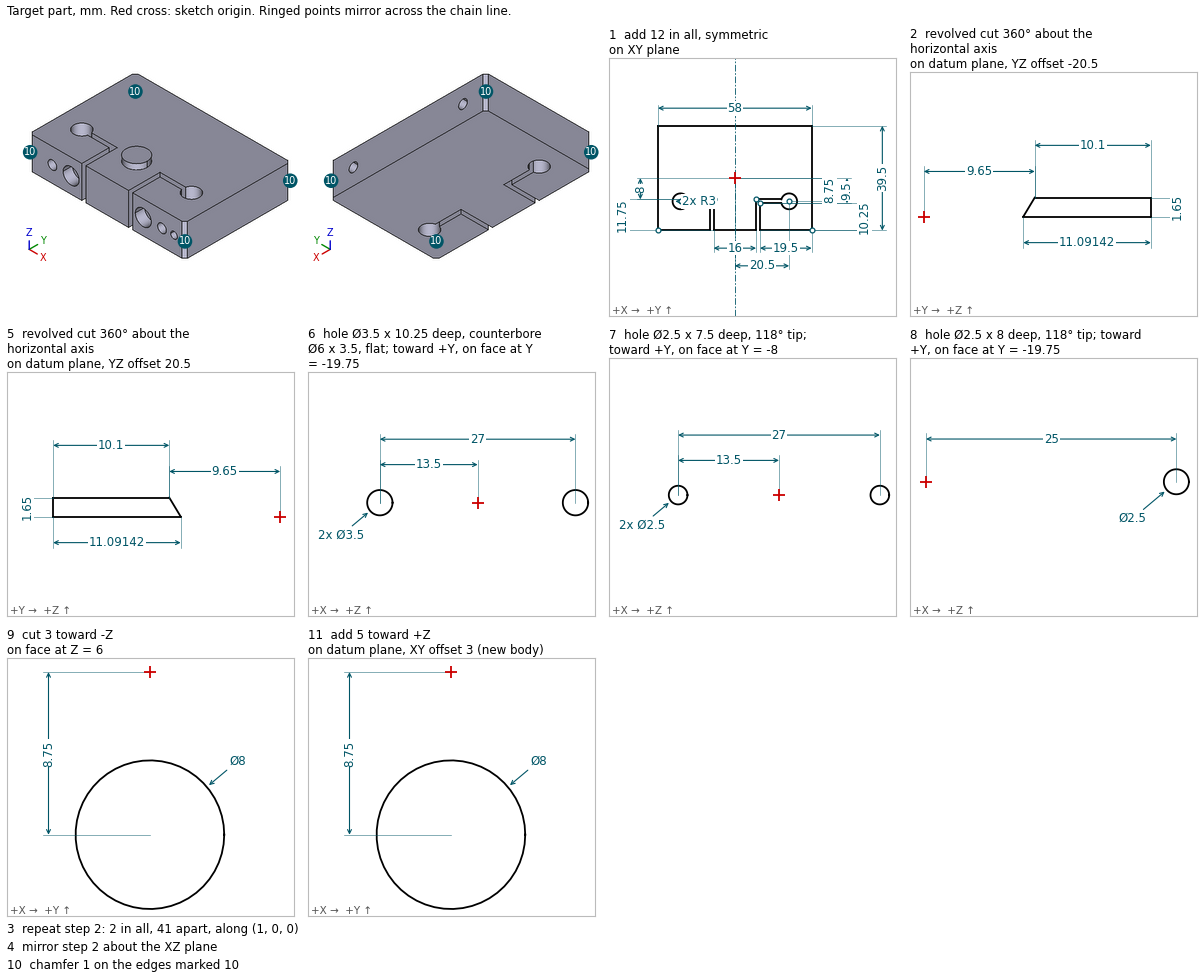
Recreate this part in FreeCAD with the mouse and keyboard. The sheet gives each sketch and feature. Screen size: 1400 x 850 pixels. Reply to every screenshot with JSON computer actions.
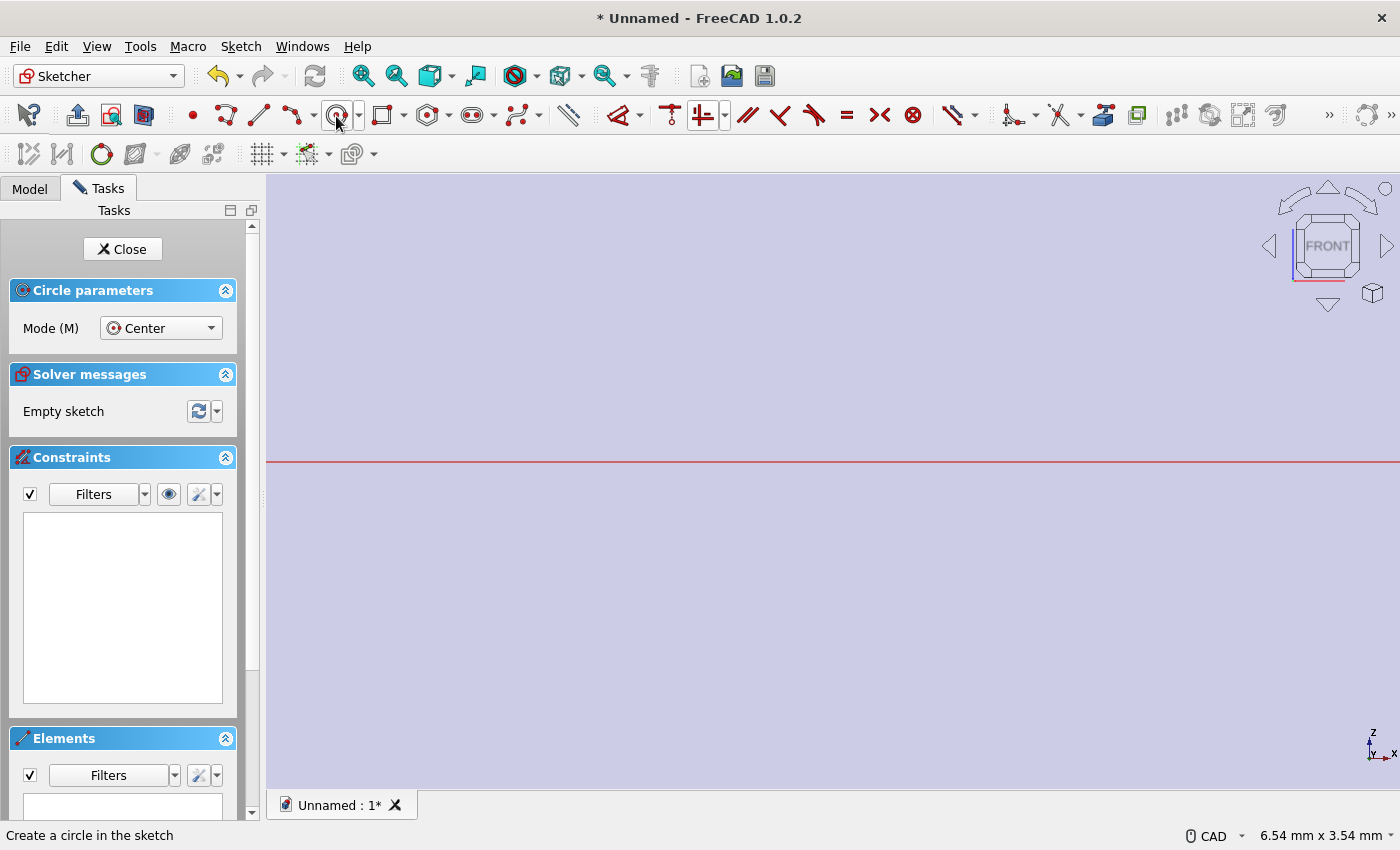
{"action": "left_click", "coordinate": [749, 462]}
{"action": "left_click", "coordinate": [902, 309]}
{"action": "key", "text": "Escape"}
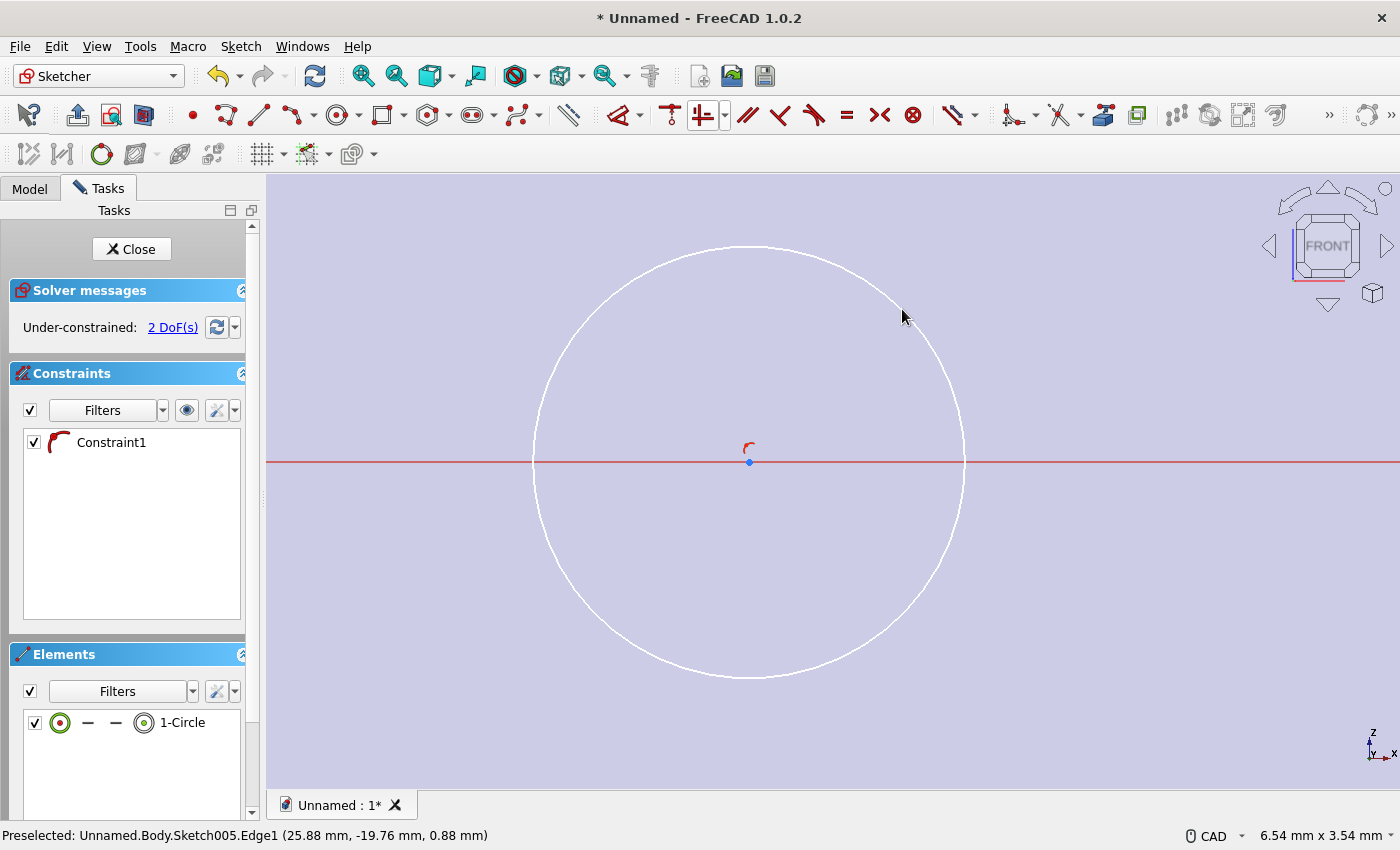
{"action": "left_click", "coordinate": [618, 116]}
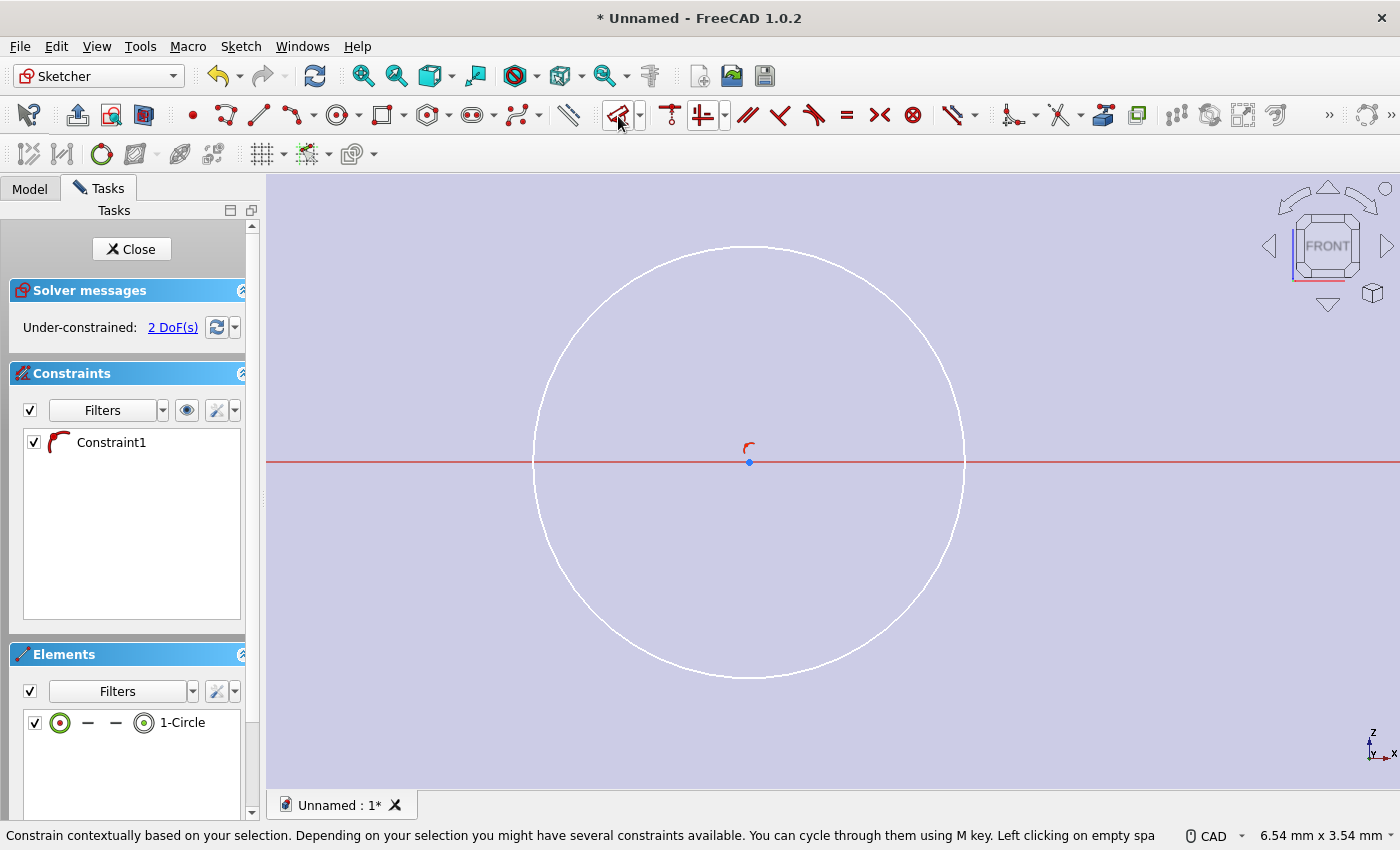
{"action": "left_click", "coordinate": [901, 309]}
{"action": "left_click", "coordinate": [924, 286]}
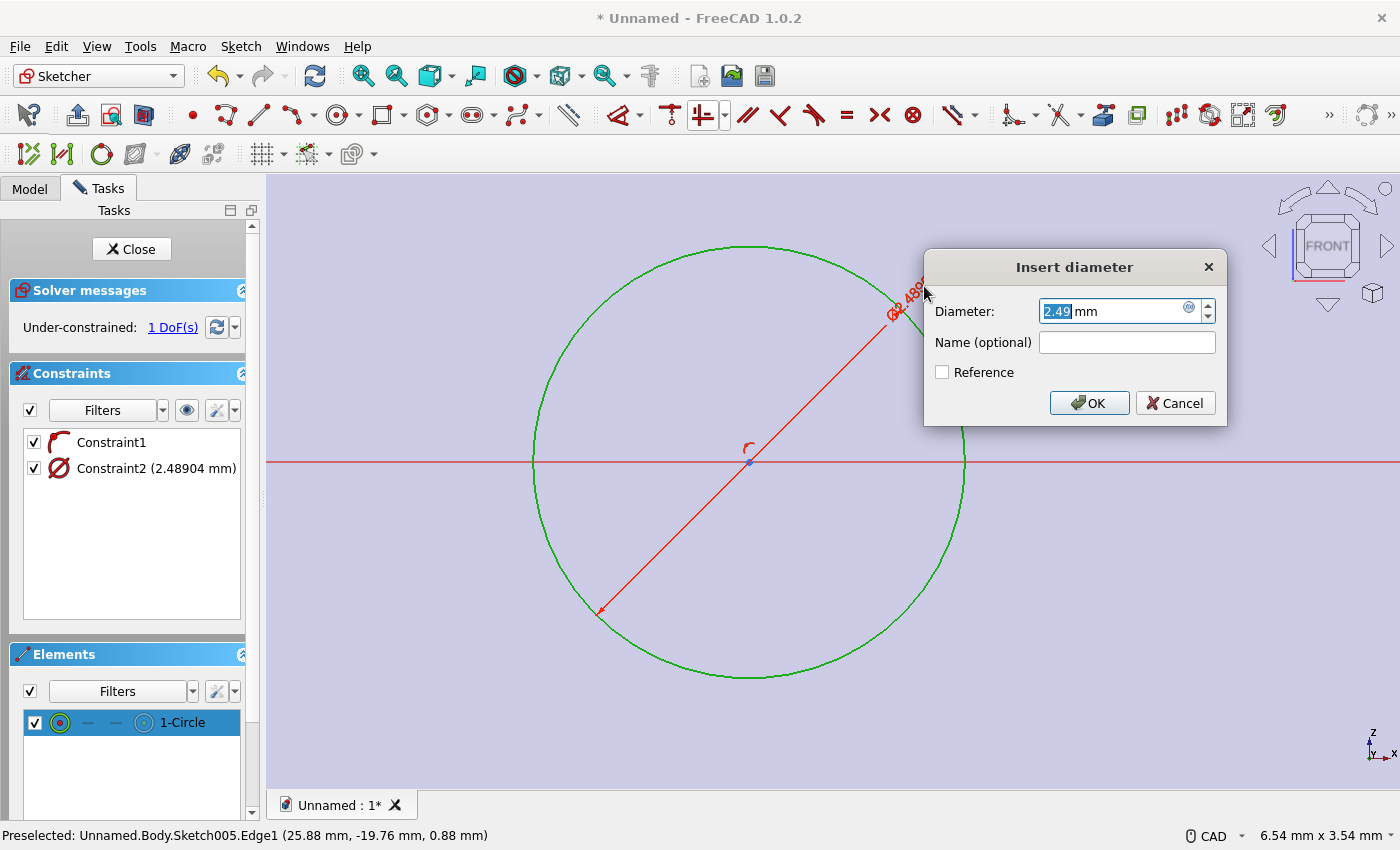
{"action": "type", "text": "2.5"}
{"action": "key", "text": "Return"}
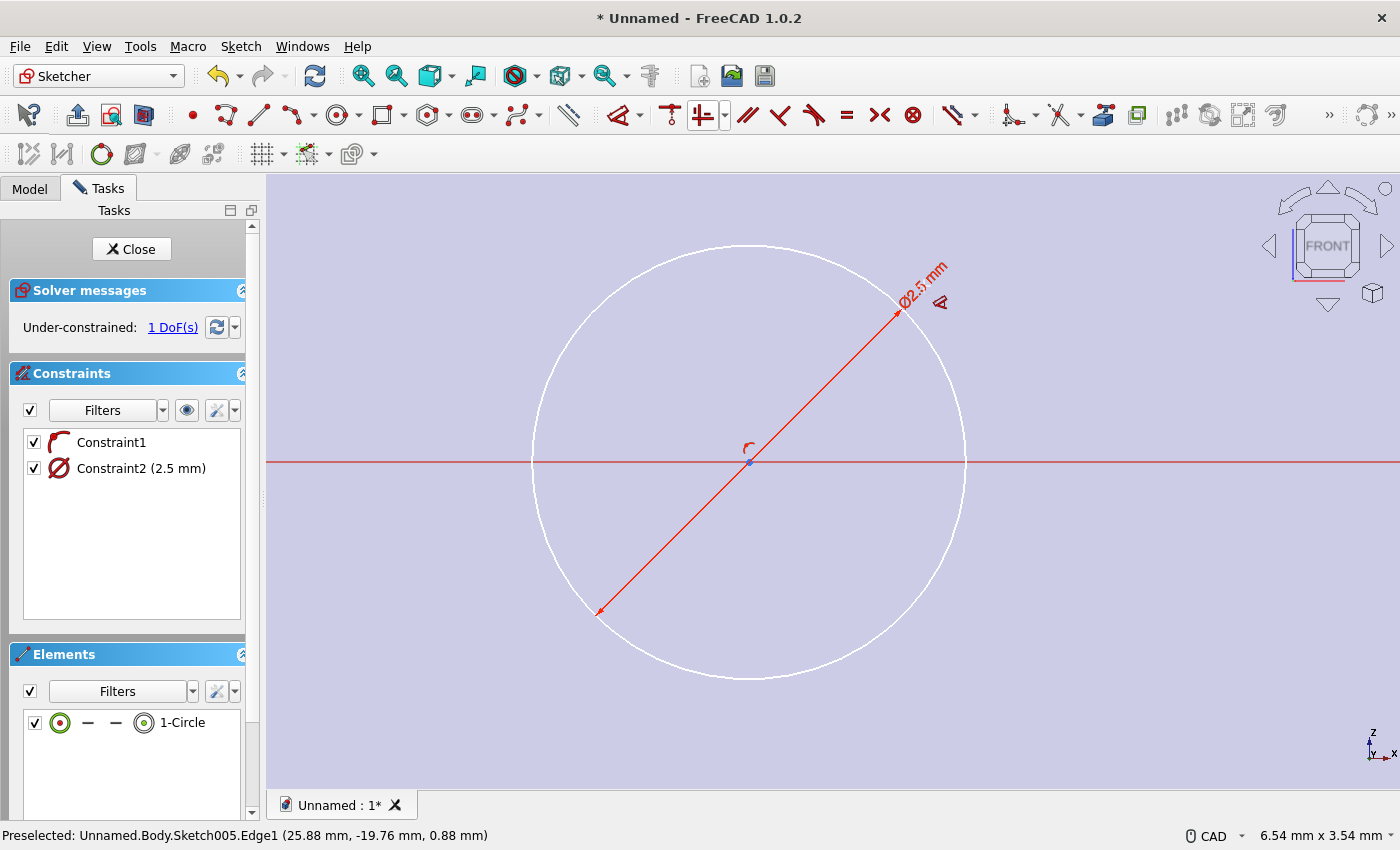
{"action": "left_click", "coordinate": [749, 462]}
{"action": "left_click", "coordinate": [522, 496]}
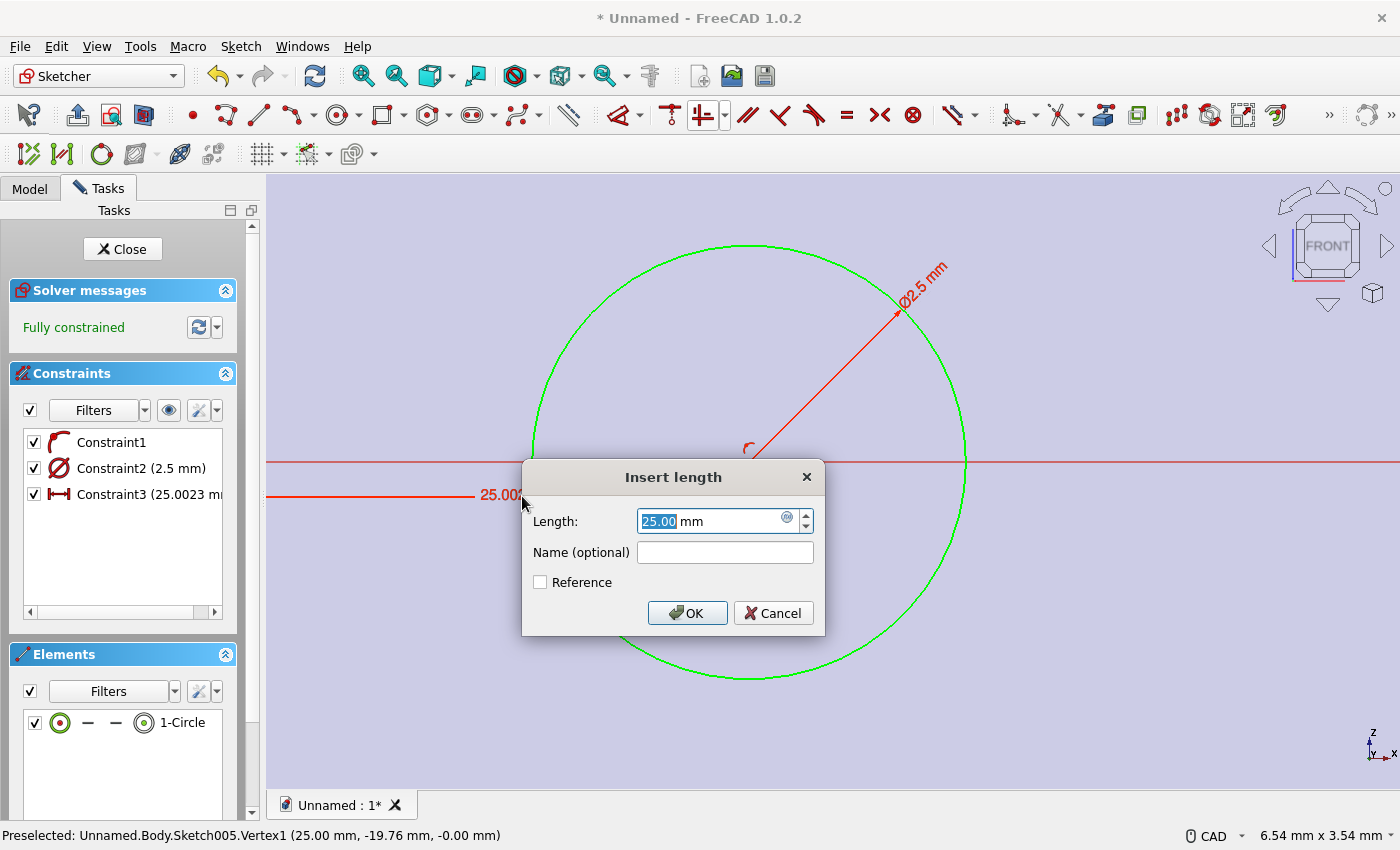
{"action": "type", "text": "25"}
{"action": "key", "text": "Return"}
{"action": "key", "text": "Escape"}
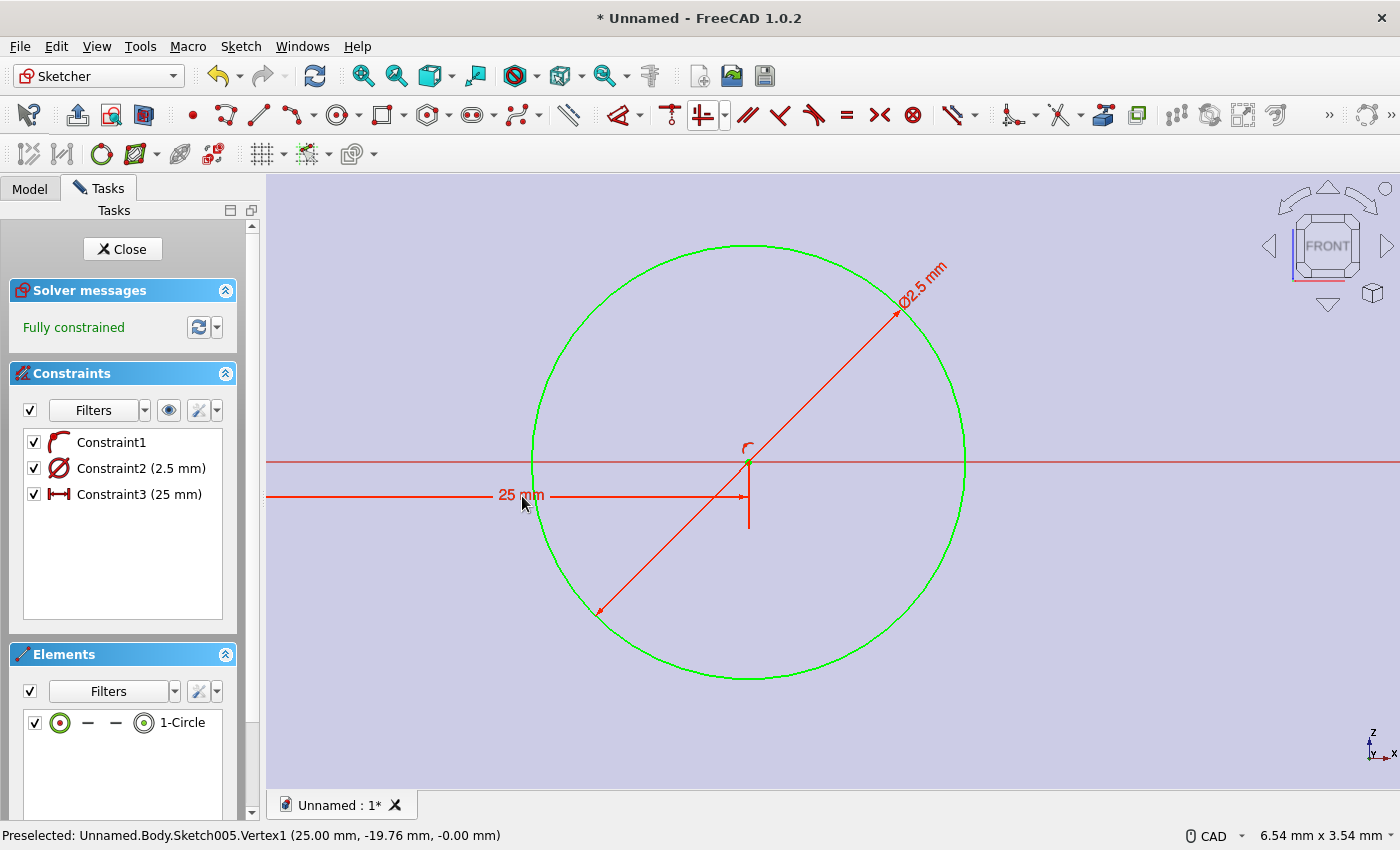
{"action": "left_click", "coordinate": [123, 249]}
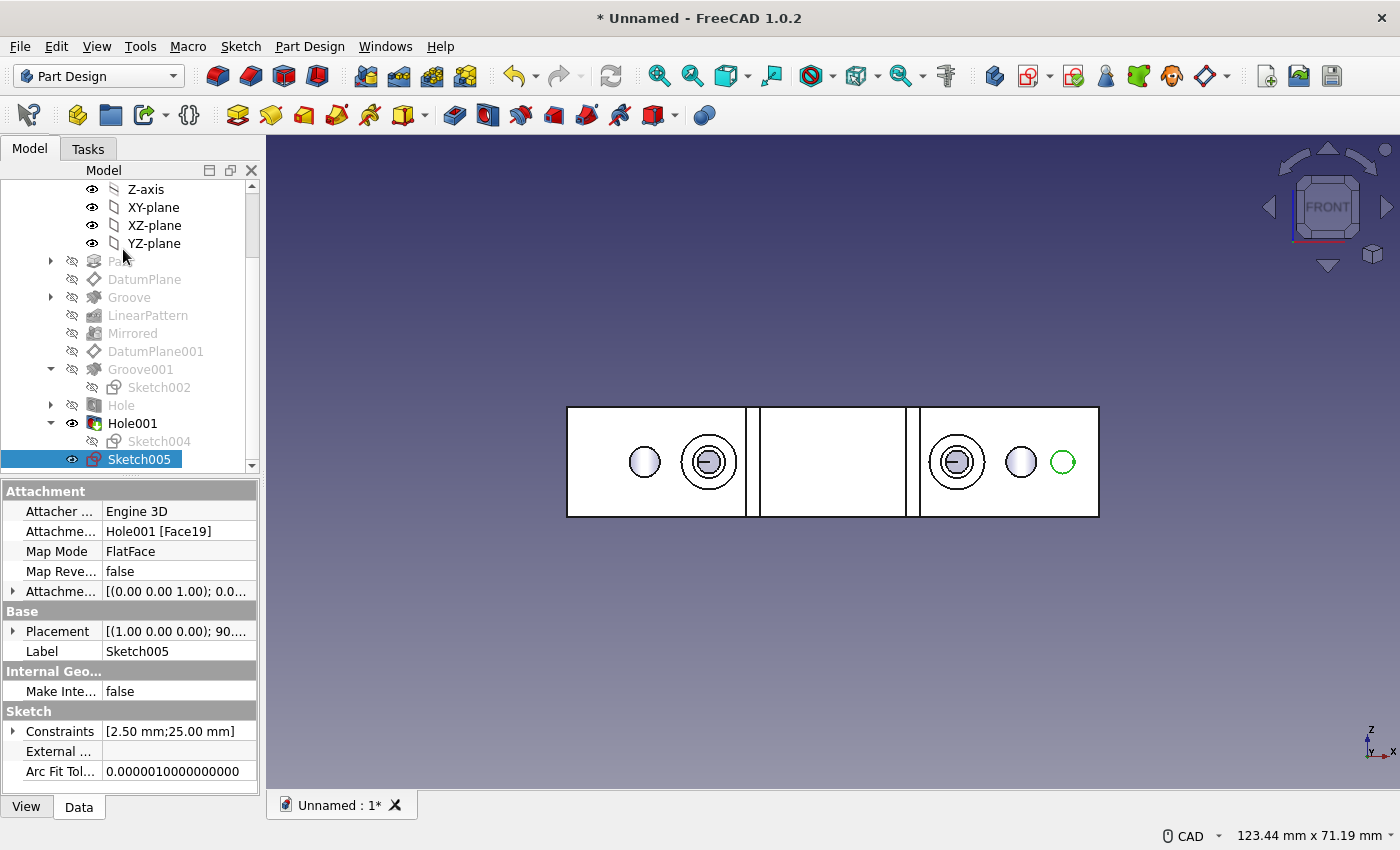
{"action": "left_click", "coordinate": [488, 116]}